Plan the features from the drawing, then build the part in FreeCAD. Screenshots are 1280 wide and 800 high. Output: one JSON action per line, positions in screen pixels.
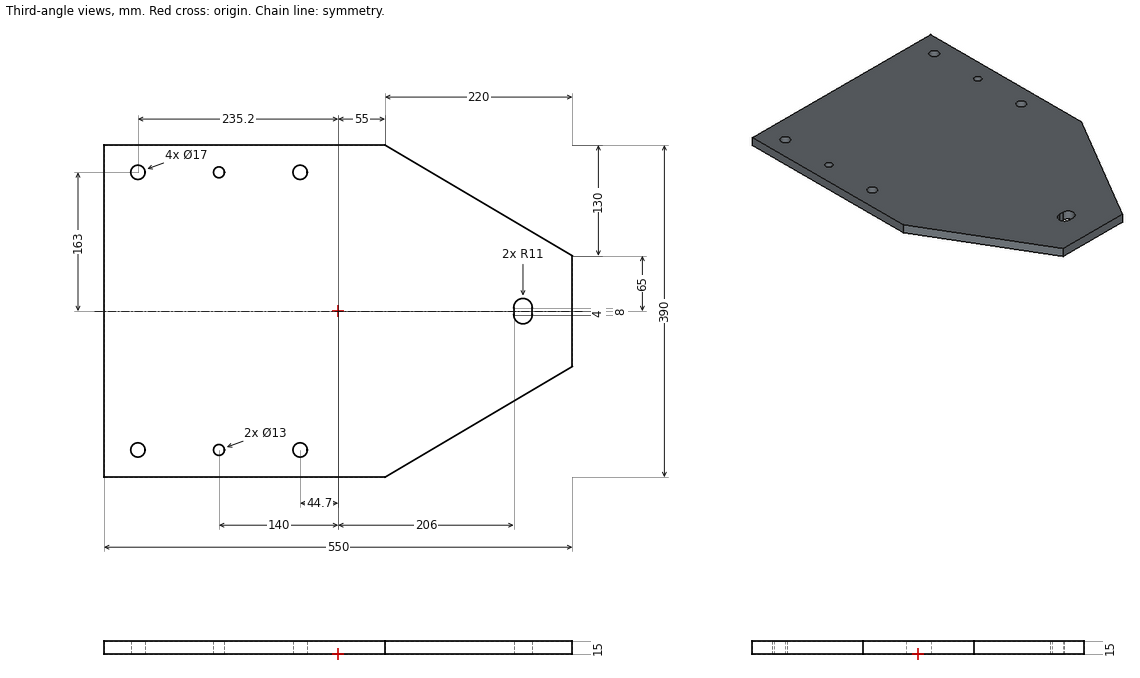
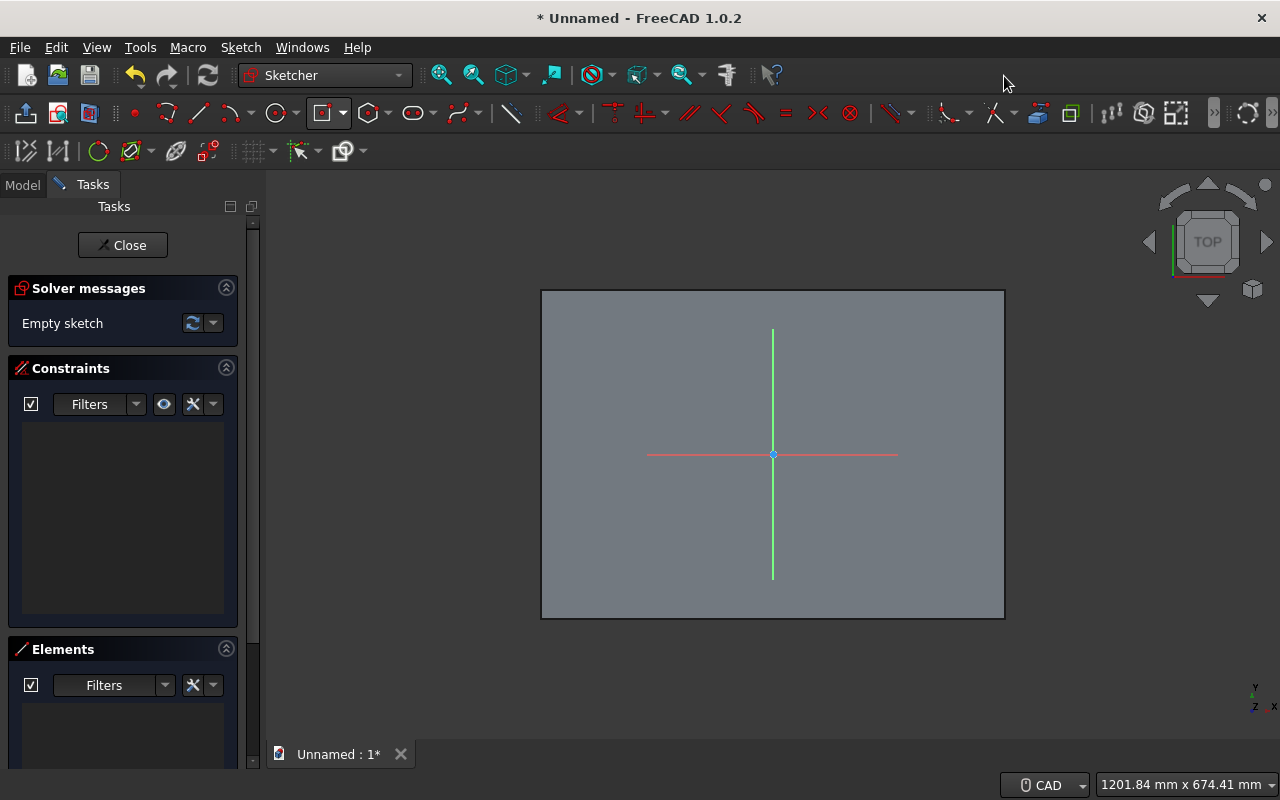
{"action": "left_click", "coordinate": [168, 114]}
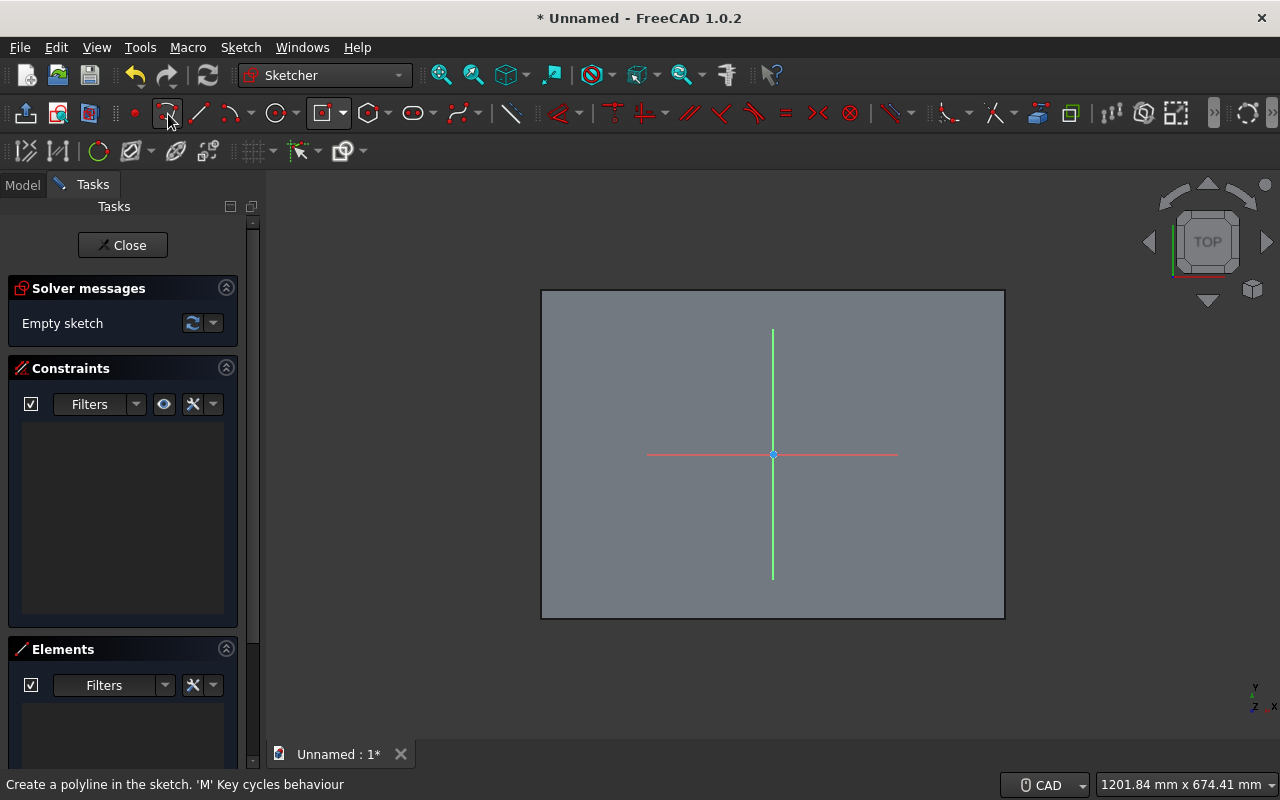
{"action": "left_click", "coordinate": [819, 290]}
{"action": "left_click", "coordinate": [1005, 400]}
{"action": "left_click", "coordinate": [1005, 290]}
{"action": "left_click", "coordinate": [819, 291]}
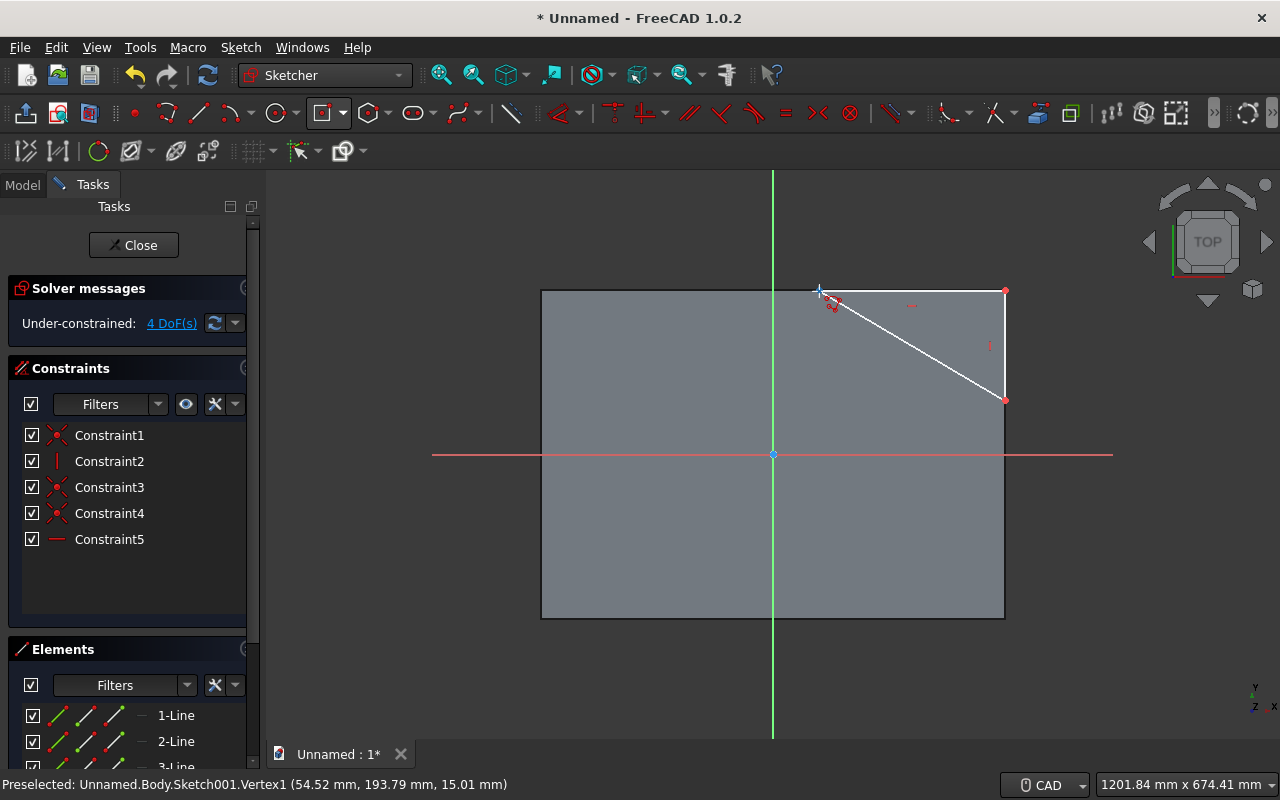
{"action": "left_click", "coordinate": [819, 619]}
{"action": "left_click", "coordinate": [1005, 619]}
{"action": "left_click", "coordinate": [1005, 509]}
{"action": "left_click", "coordinate": [819, 620]}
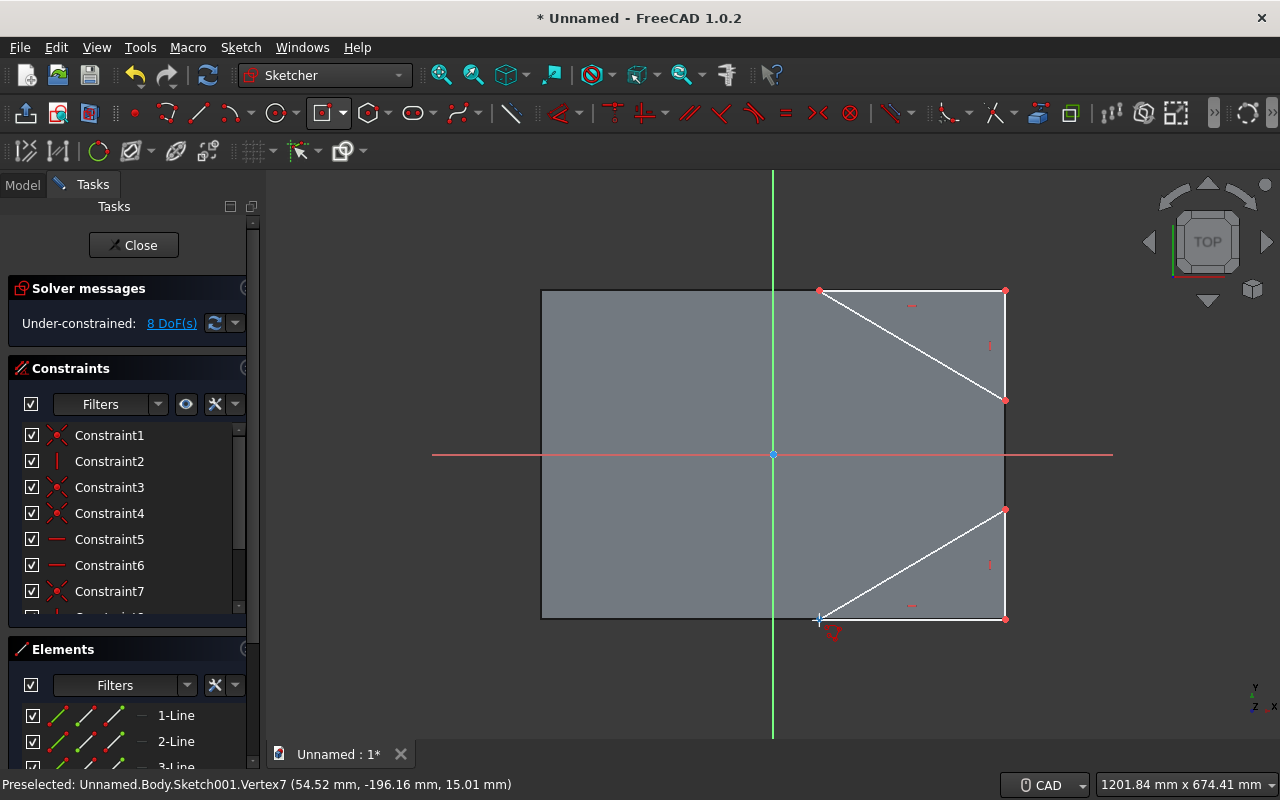
{"action": "left_click", "coordinate": [414, 114]}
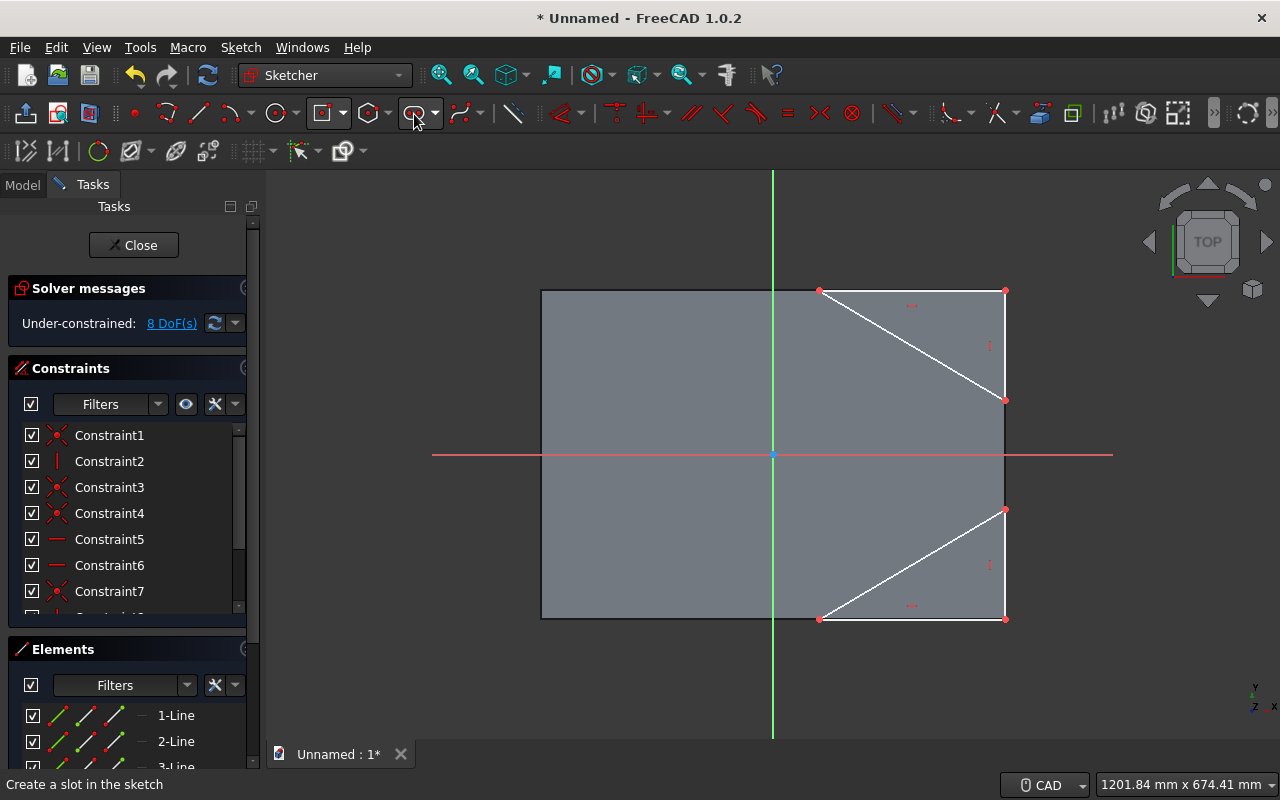
{"action": "scroll", "coordinate": [956, 458], "scroll_direction": "up", "scroll_amount": 8}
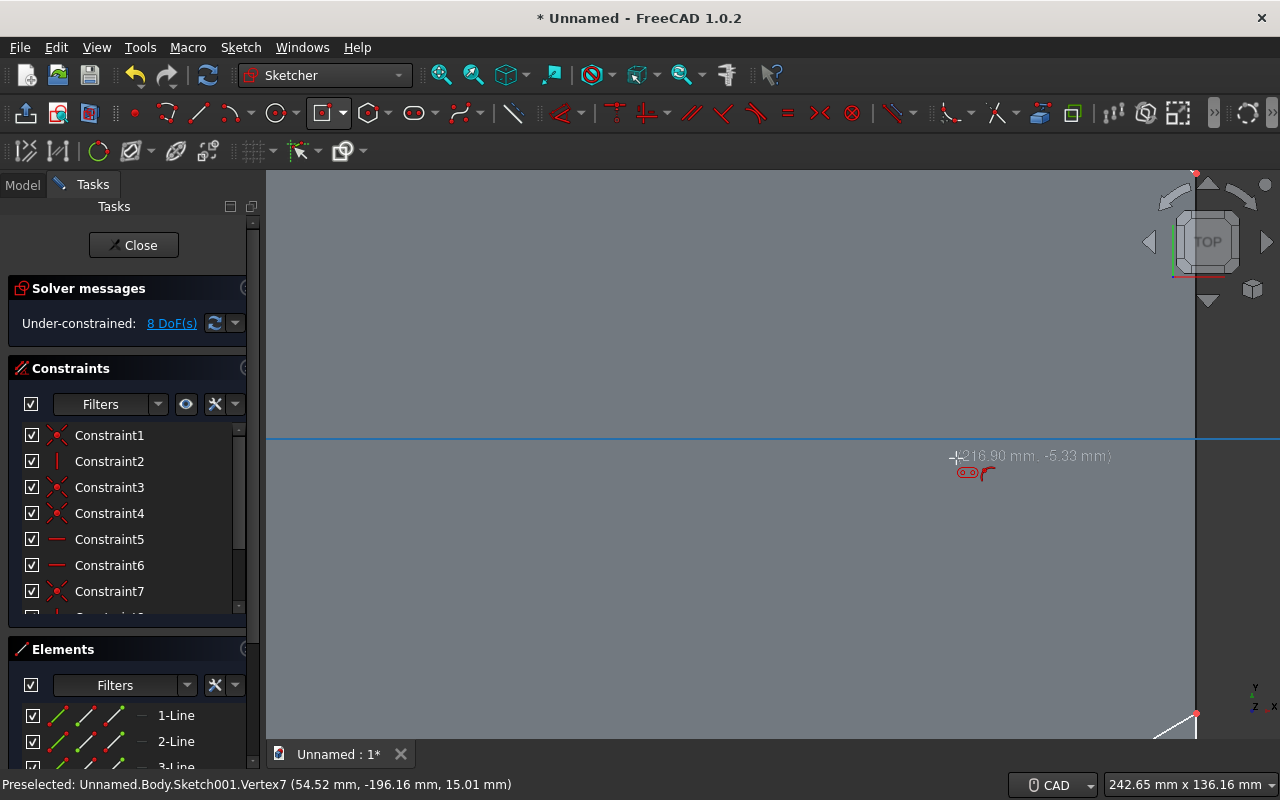
{"action": "left_click", "coordinate": [954, 455]}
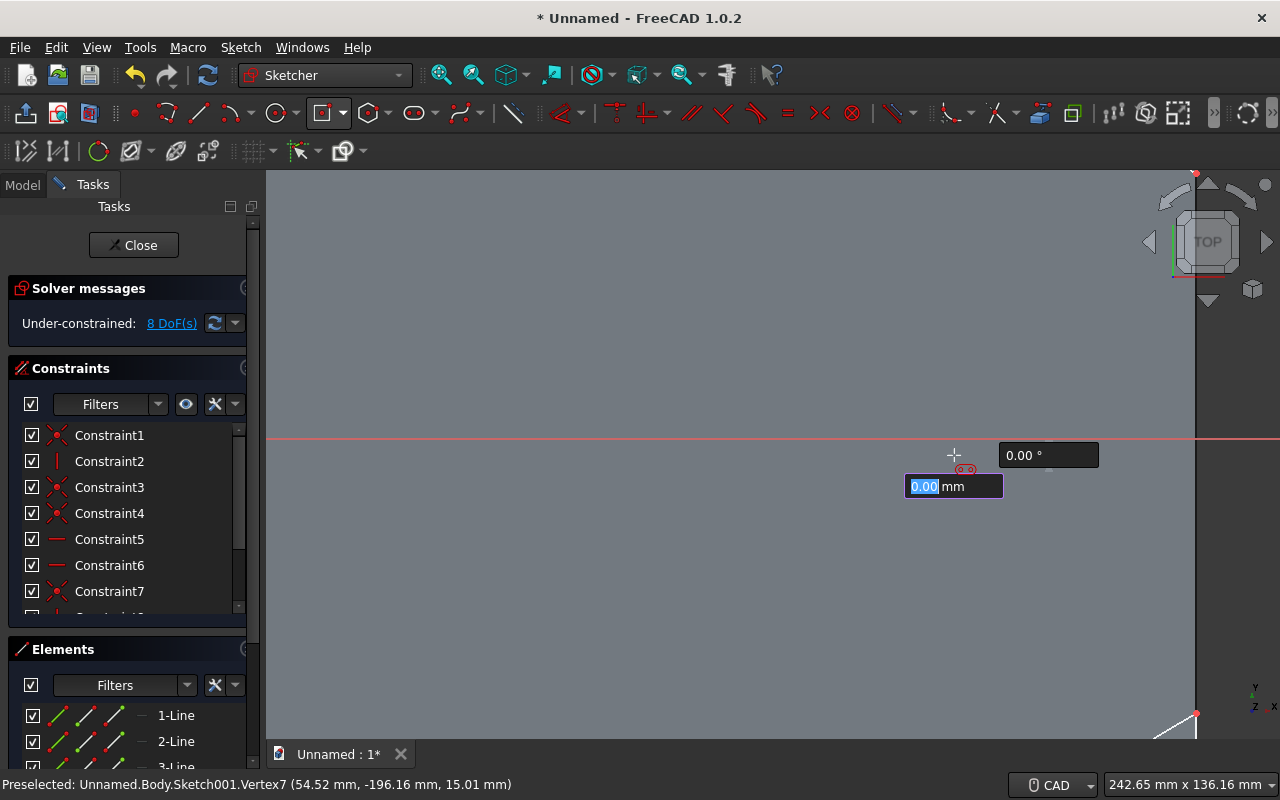
{"action": "left_click", "coordinate": [954, 422]}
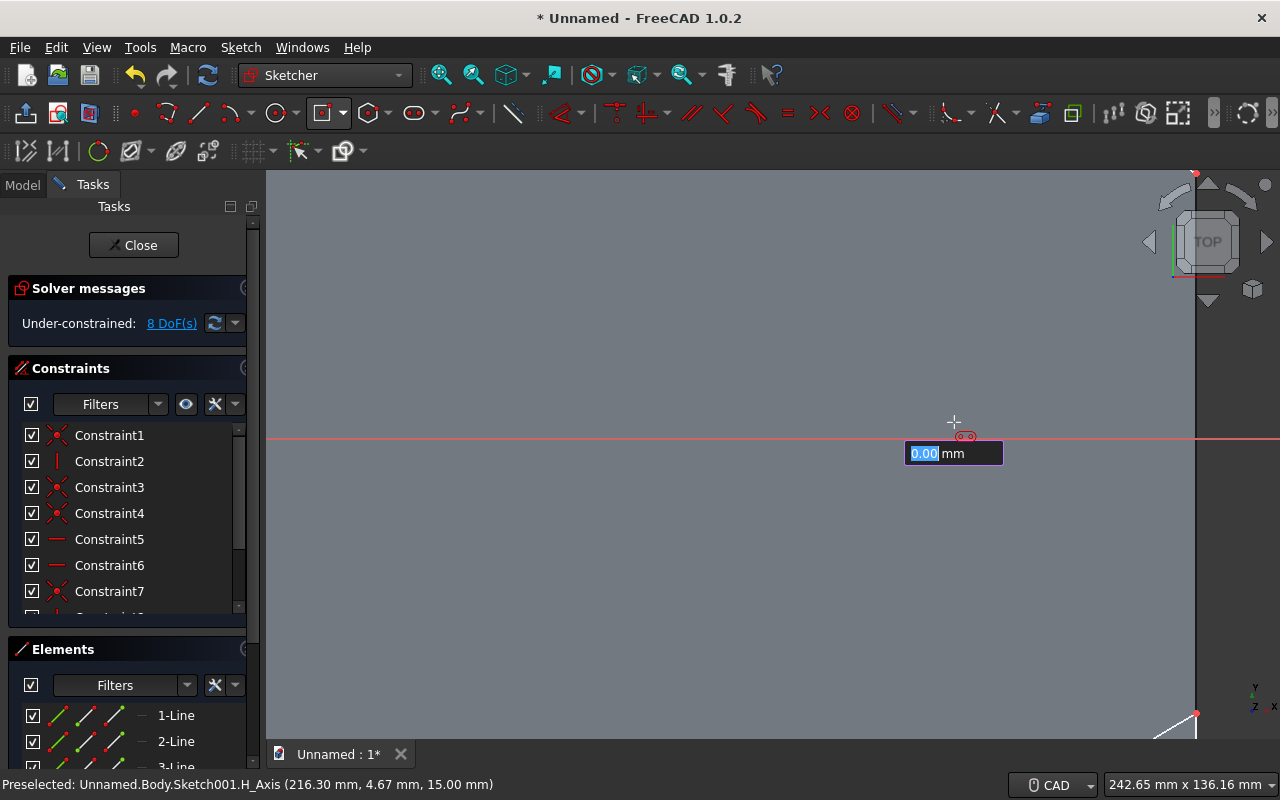
{"action": "scroll", "coordinate": [1000, 444], "scroll_direction": "up", "scroll_amount": 6}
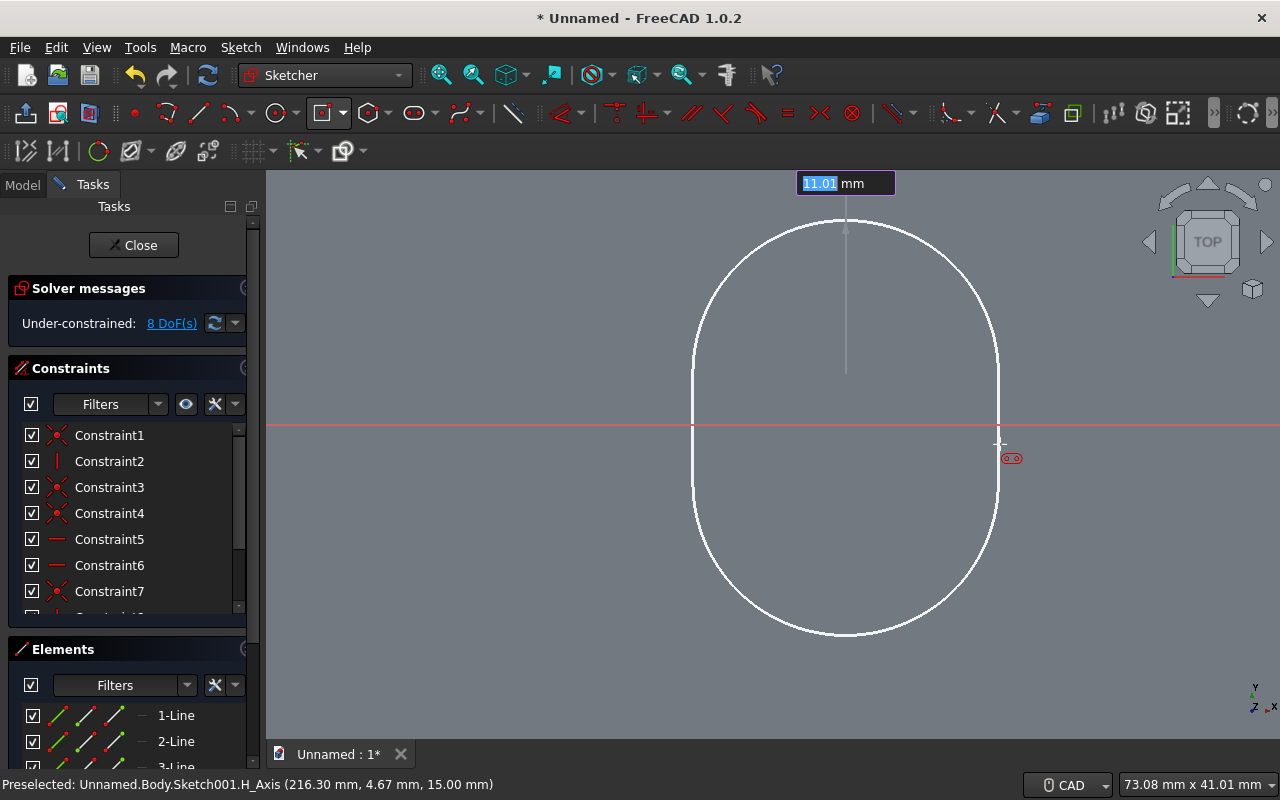
{"action": "left_click", "coordinate": [997, 442]}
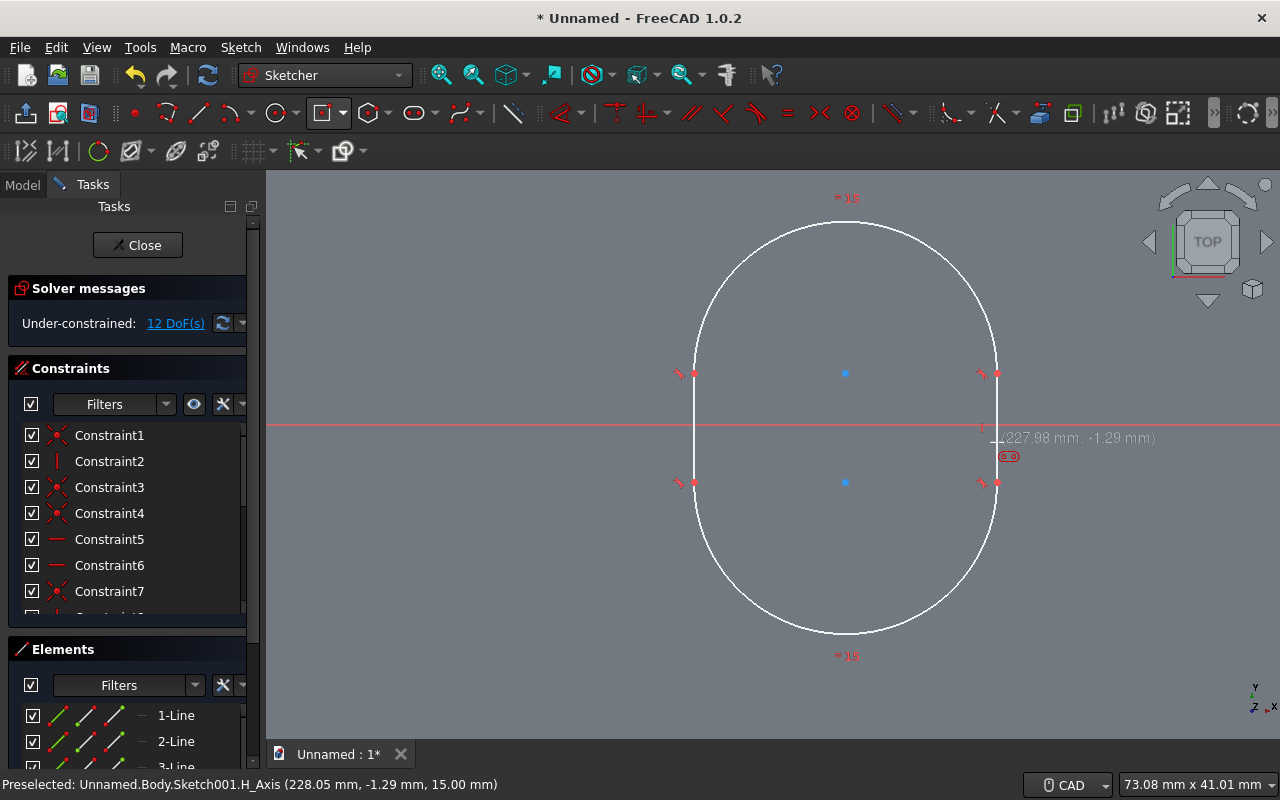
{"action": "left_click", "coordinate": [276, 114]}